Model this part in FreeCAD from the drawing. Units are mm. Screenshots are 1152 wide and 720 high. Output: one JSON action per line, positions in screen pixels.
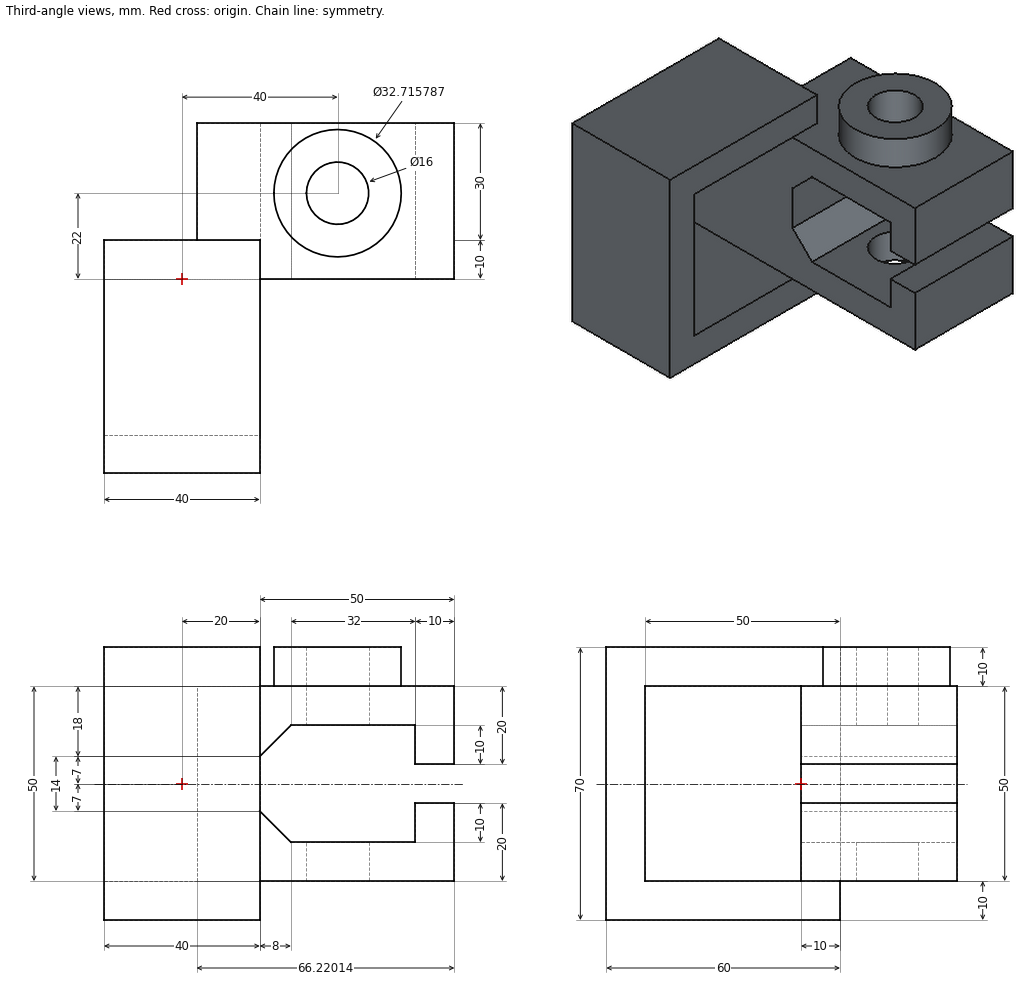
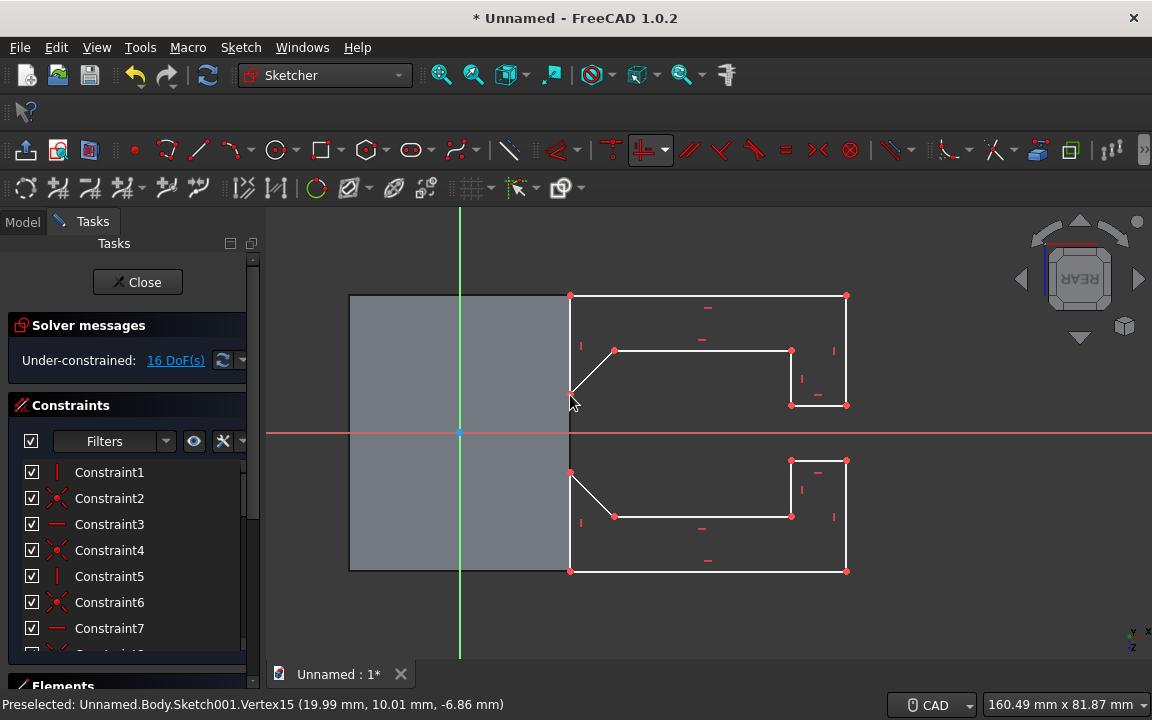
{"action": "left_click", "coordinate": [570, 473]}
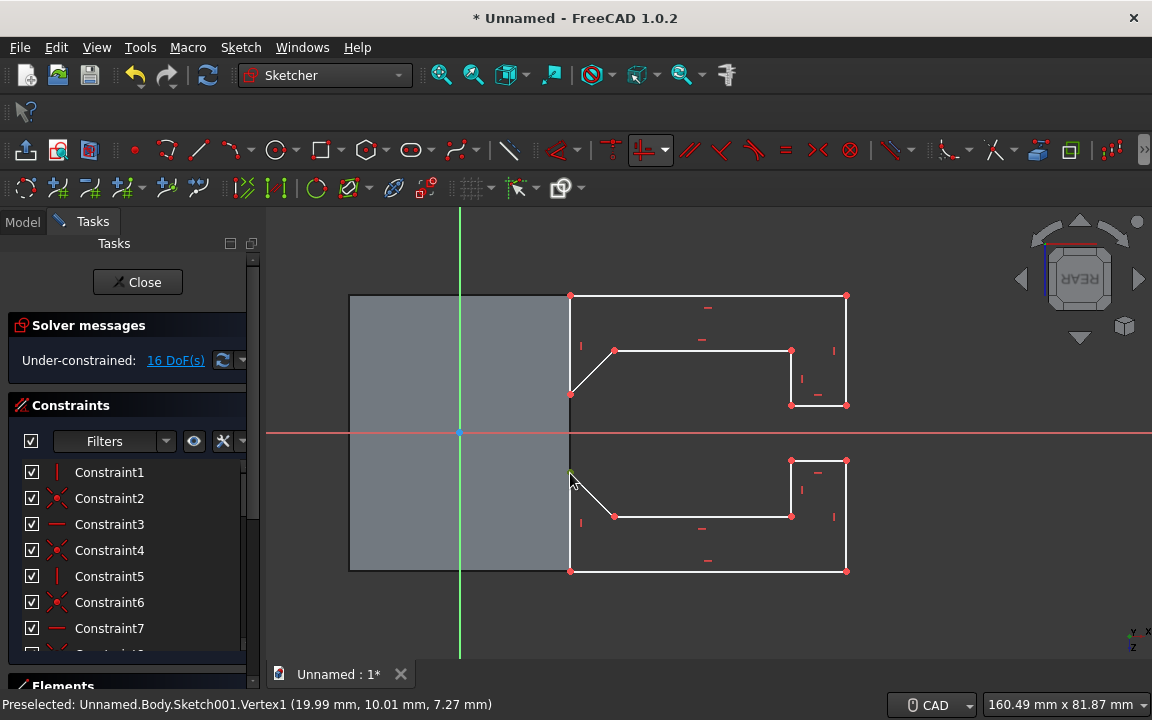
{"action": "left_click", "coordinate": [570, 395]}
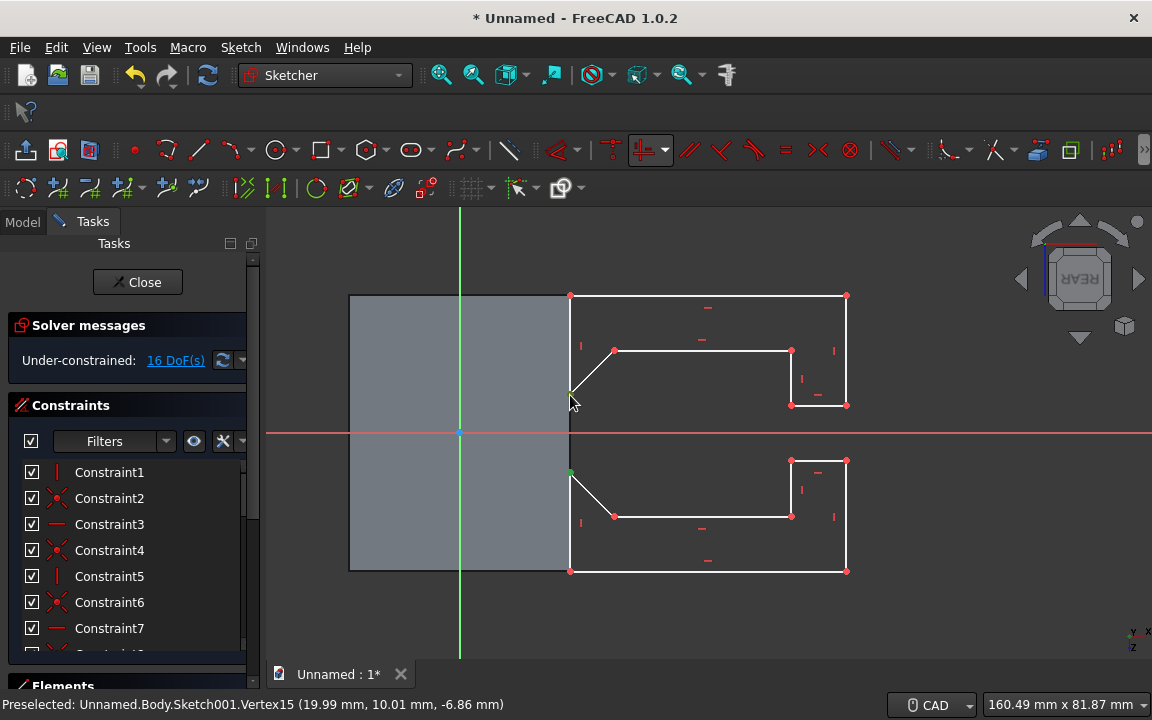
{"action": "left_click", "coordinate": [344, 433]}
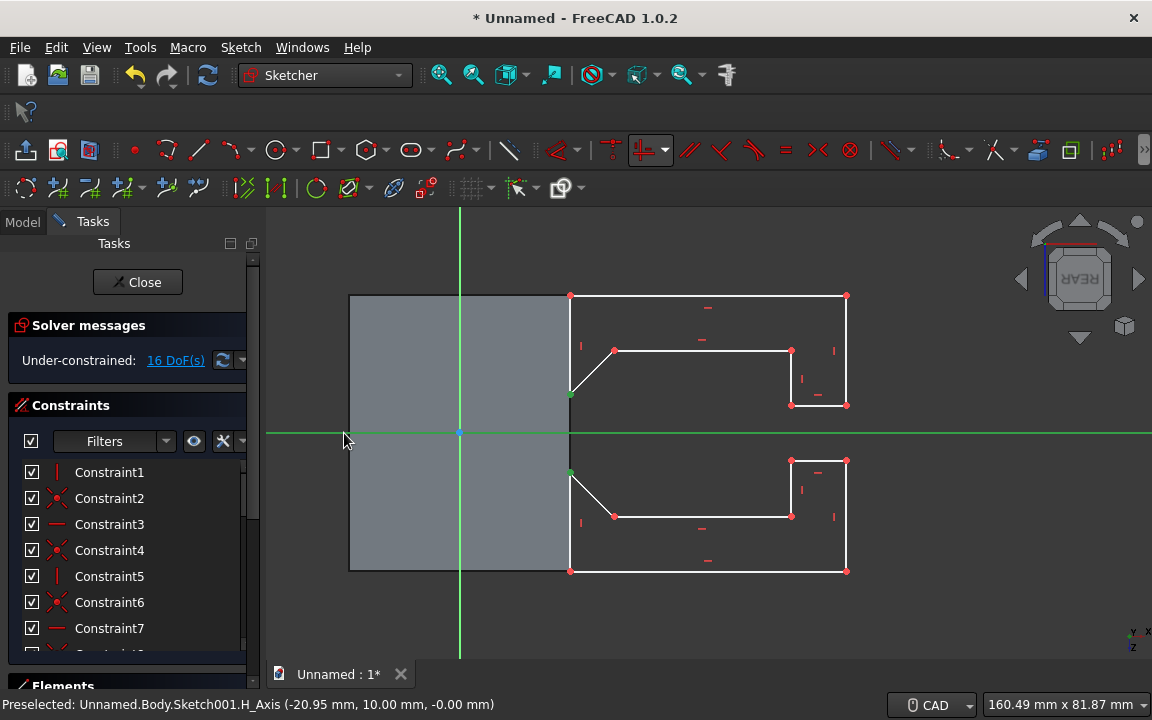
{"action": "key", "text": "s"}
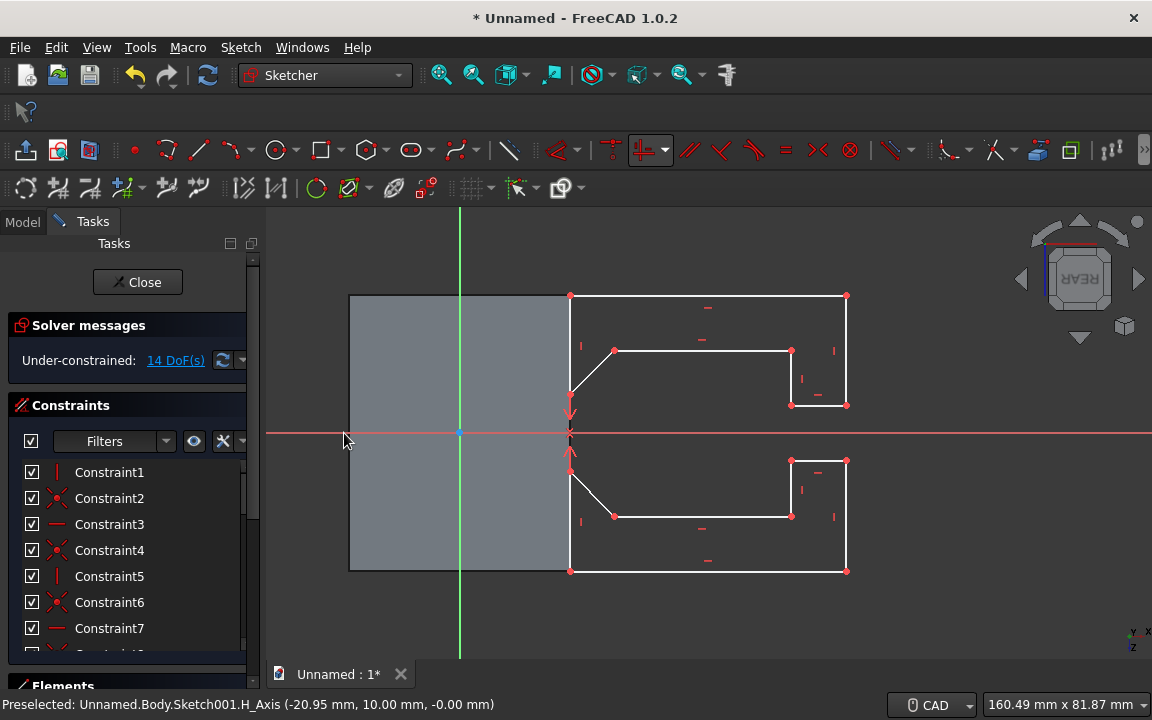
{"action": "left_click", "coordinate": [614, 517]}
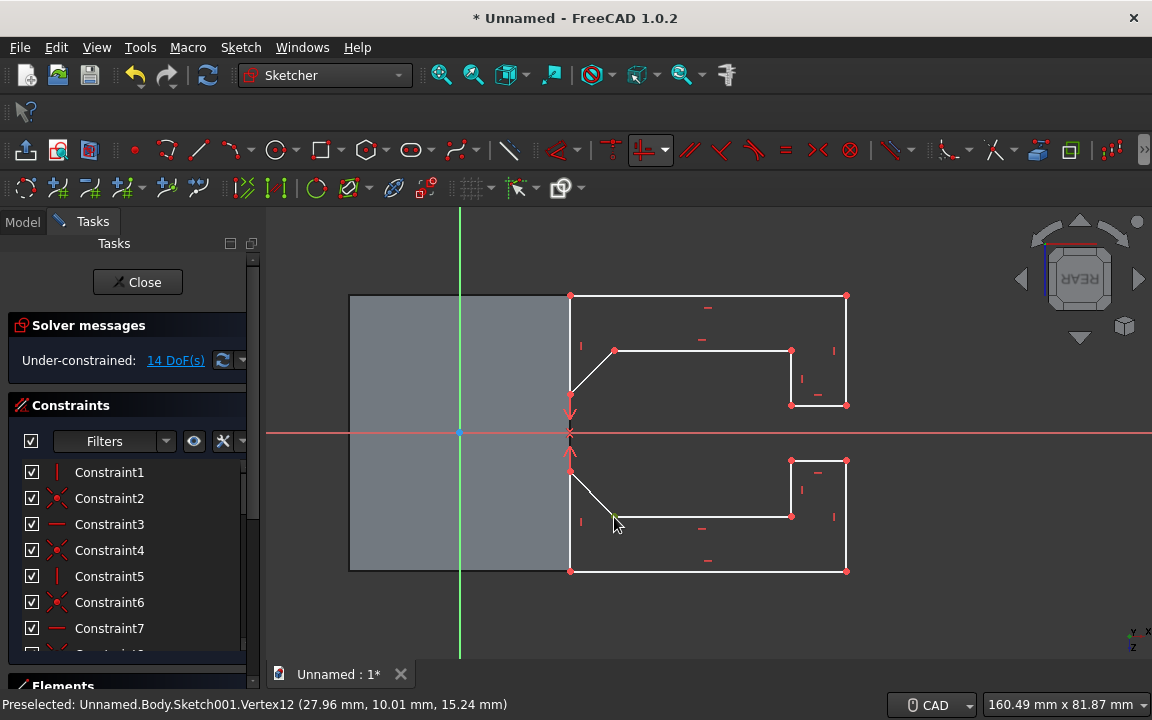
{"action": "left_click", "coordinate": [614, 351]}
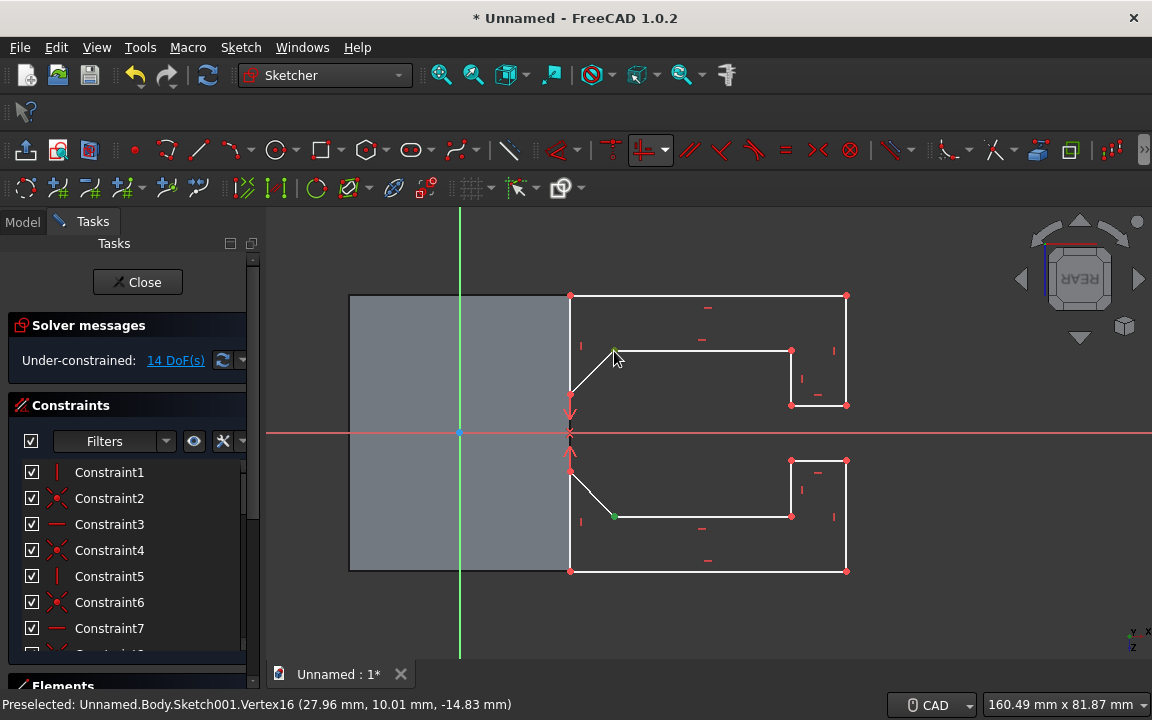
{"action": "left_click", "coordinate": [344, 433]}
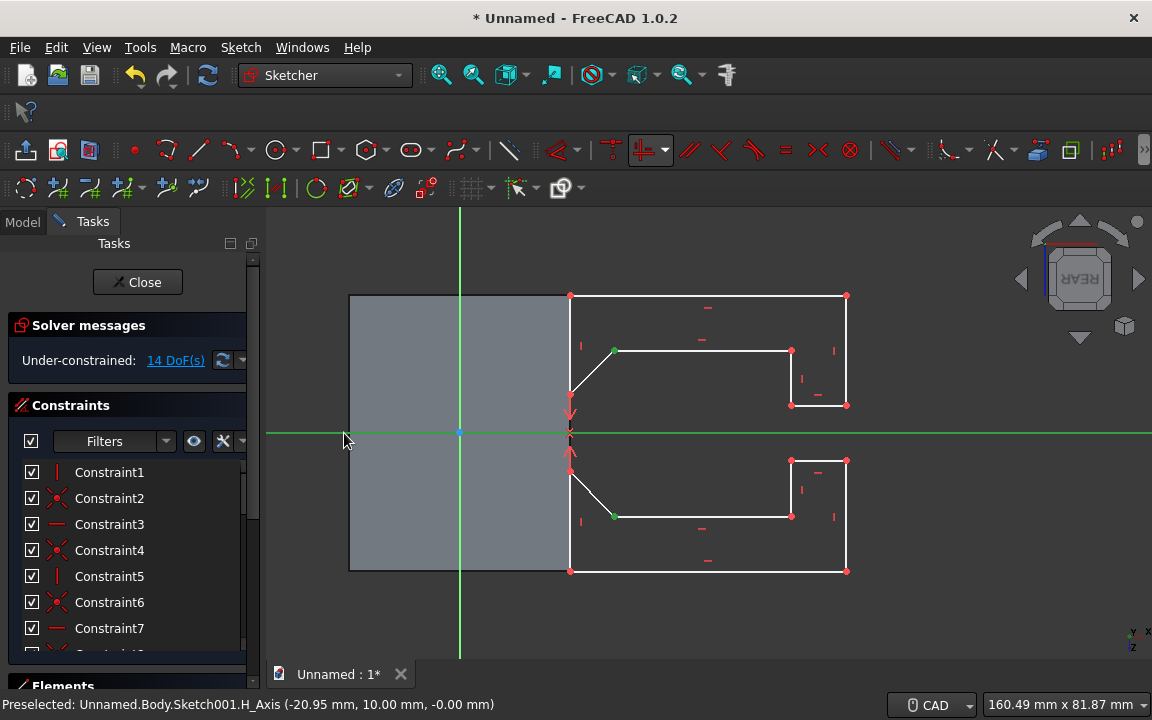
{"action": "left_click", "coordinate": [818, 150]}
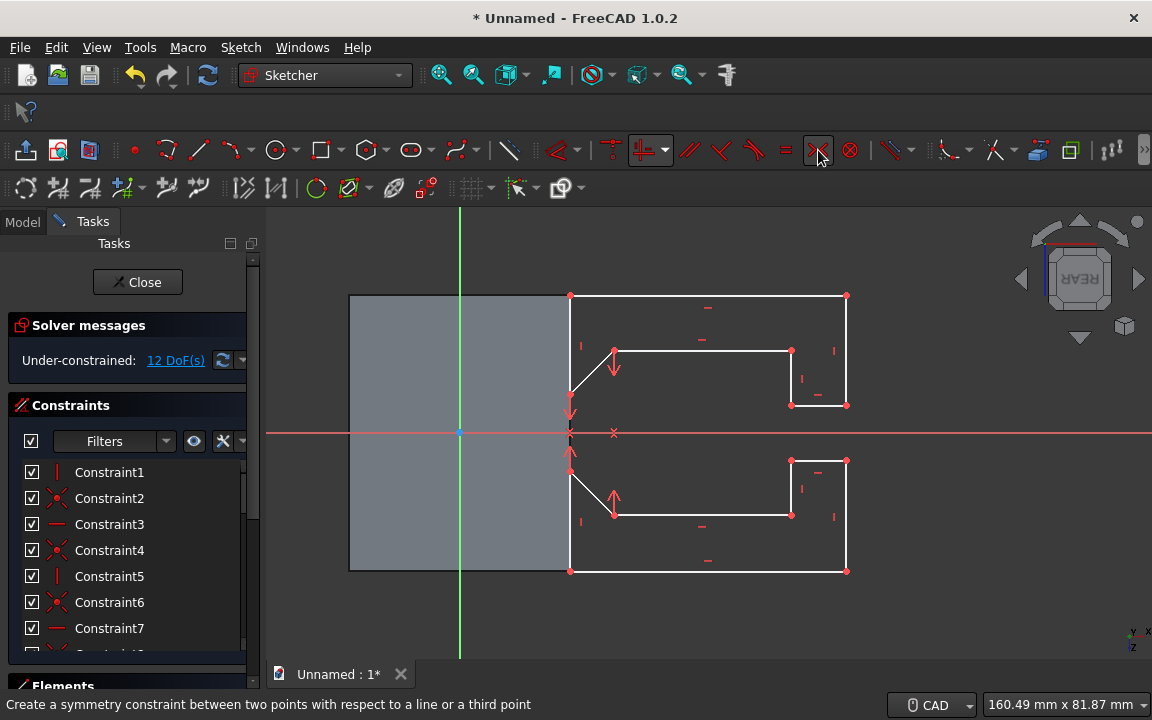
{"action": "left_click", "coordinate": [791, 461]}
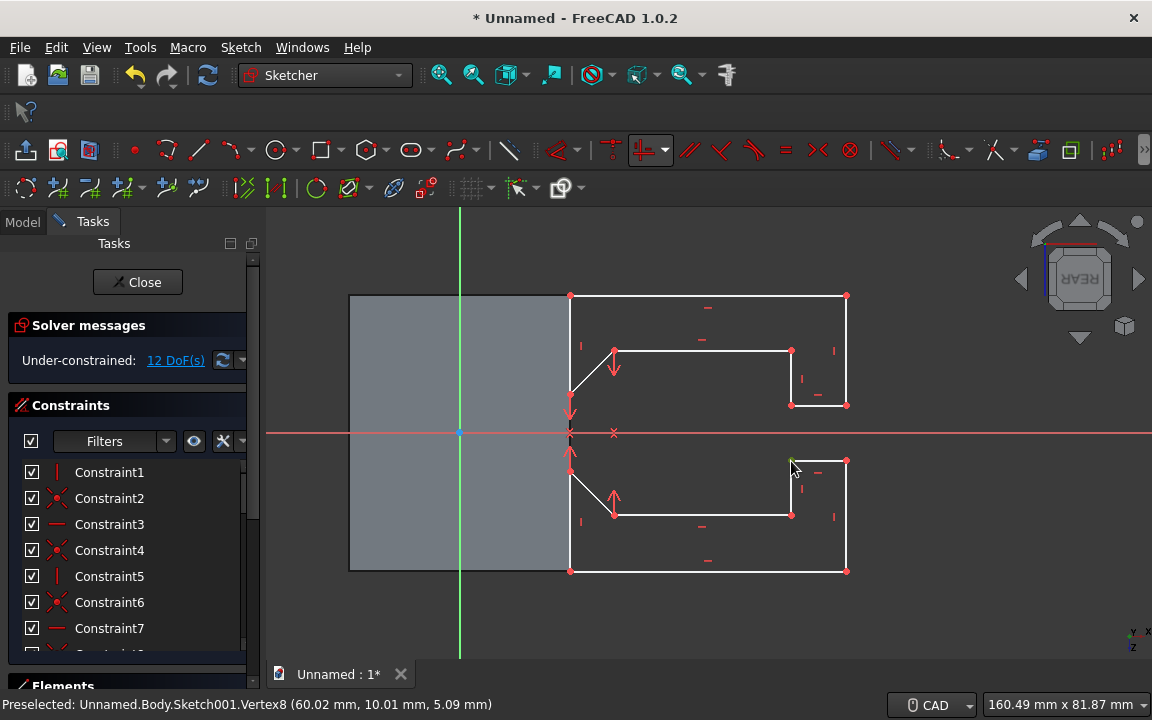
{"action": "left_click", "coordinate": [791, 406]}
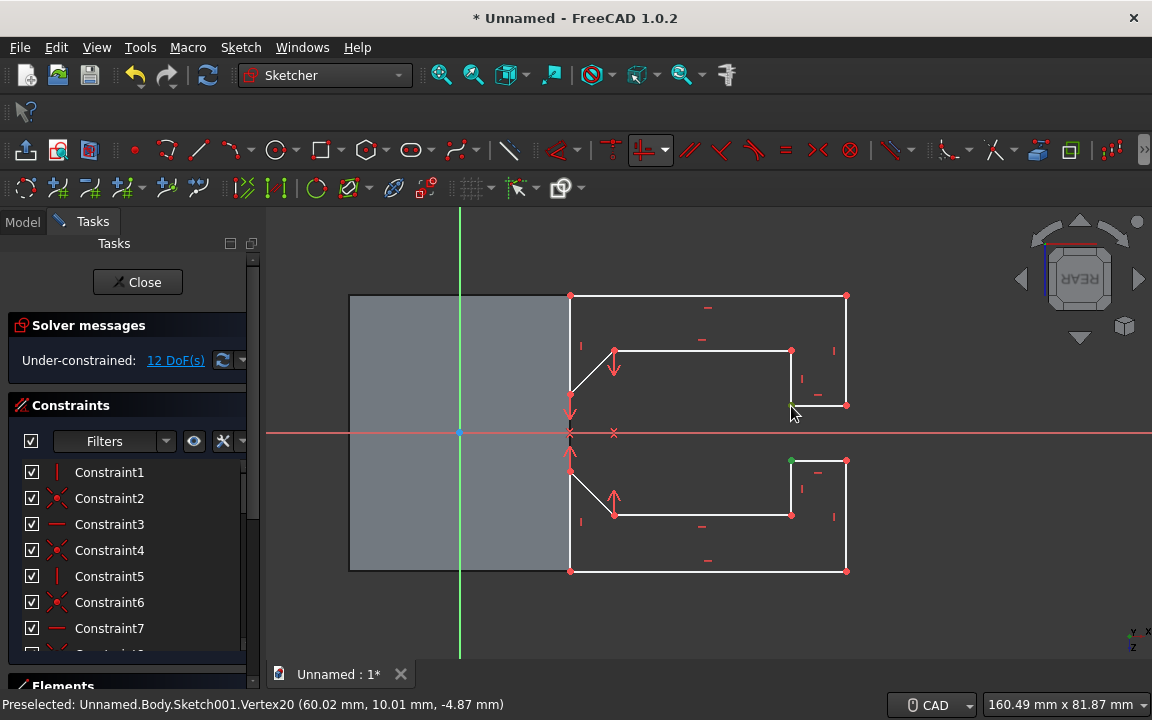
{"action": "left_click", "coordinate": [344, 433]}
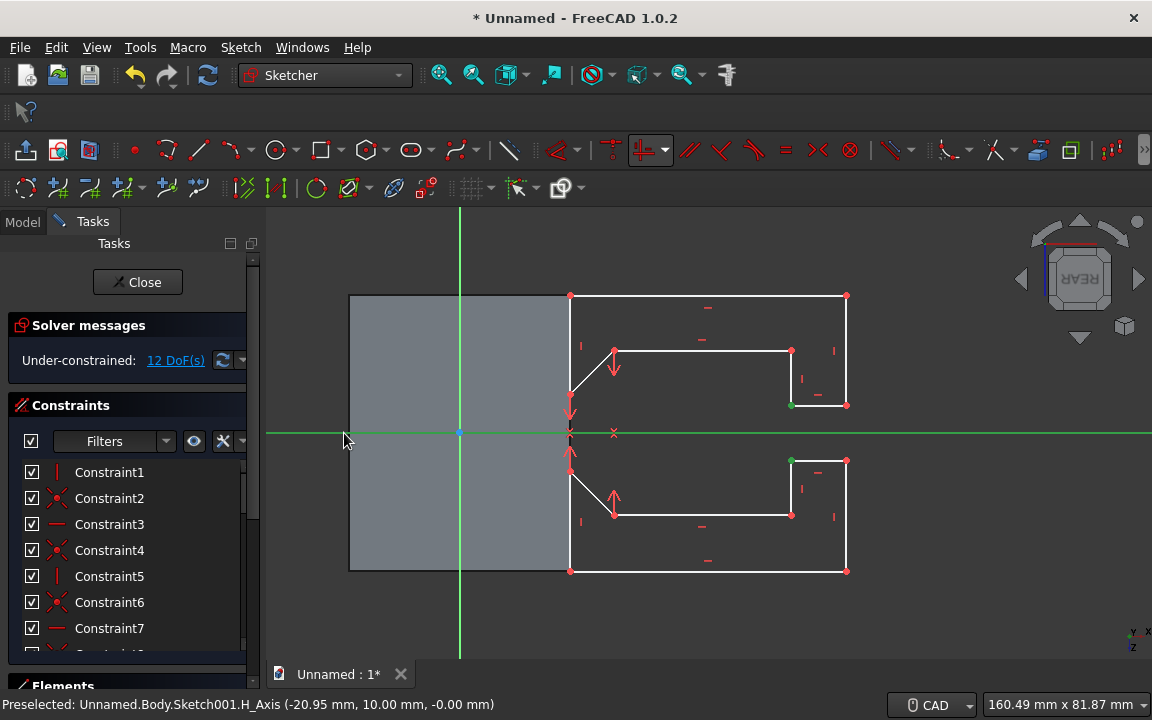
{"action": "left_click", "coordinate": [818, 150]}